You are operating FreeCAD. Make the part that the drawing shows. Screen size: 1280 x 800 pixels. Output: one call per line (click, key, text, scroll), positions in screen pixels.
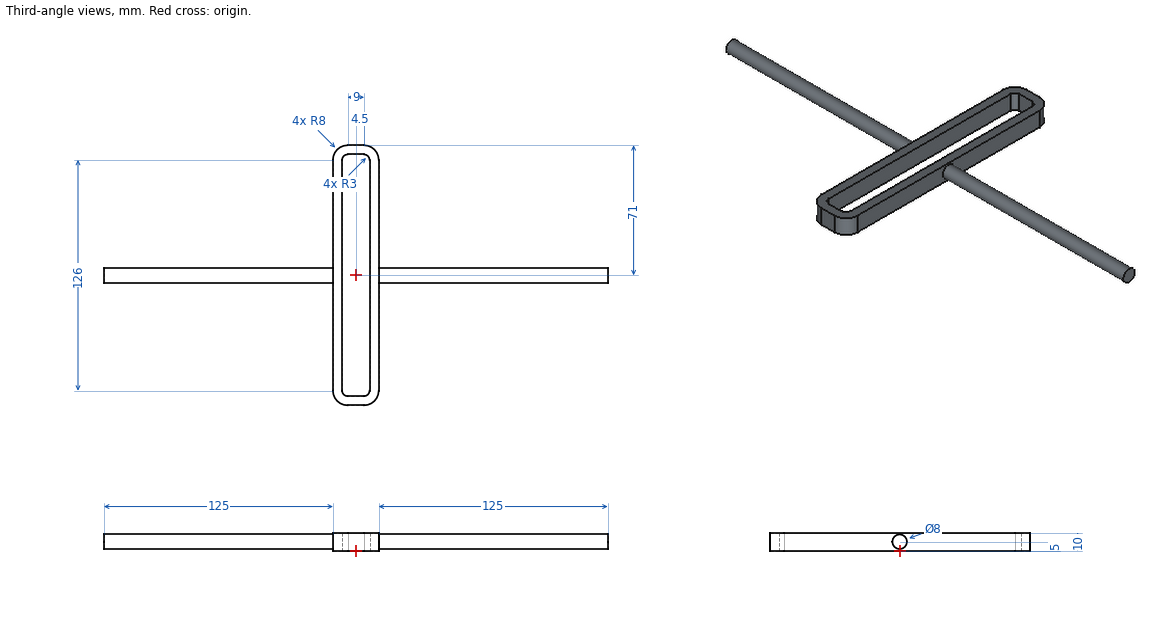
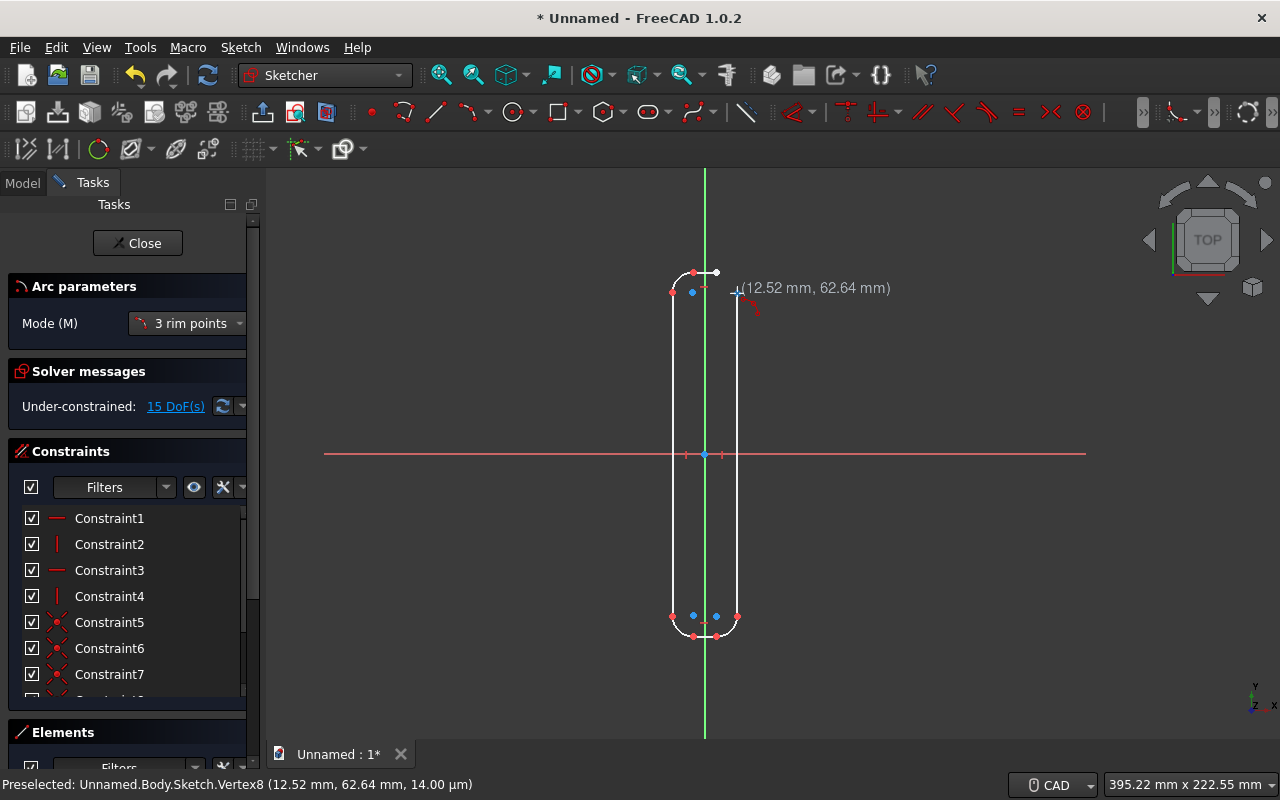
scroll(717, 272, up, 2)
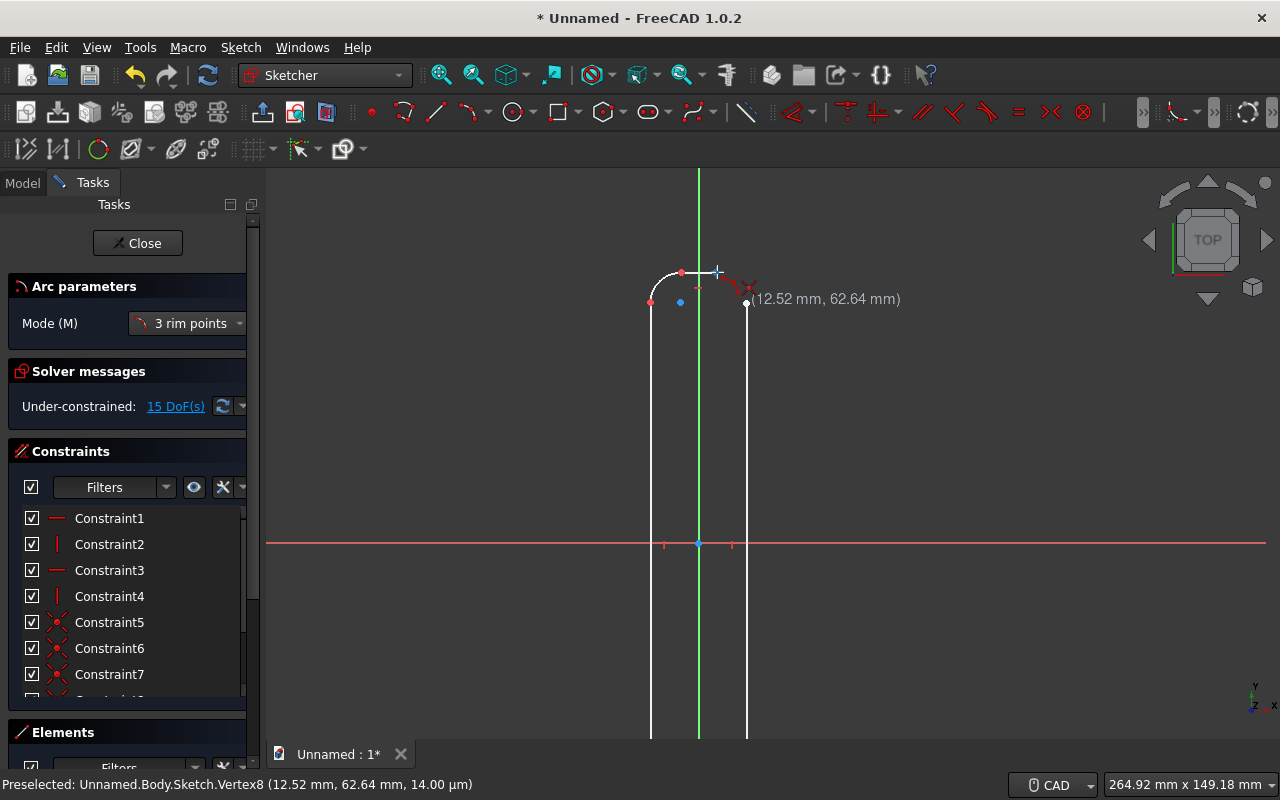
click(716, 273)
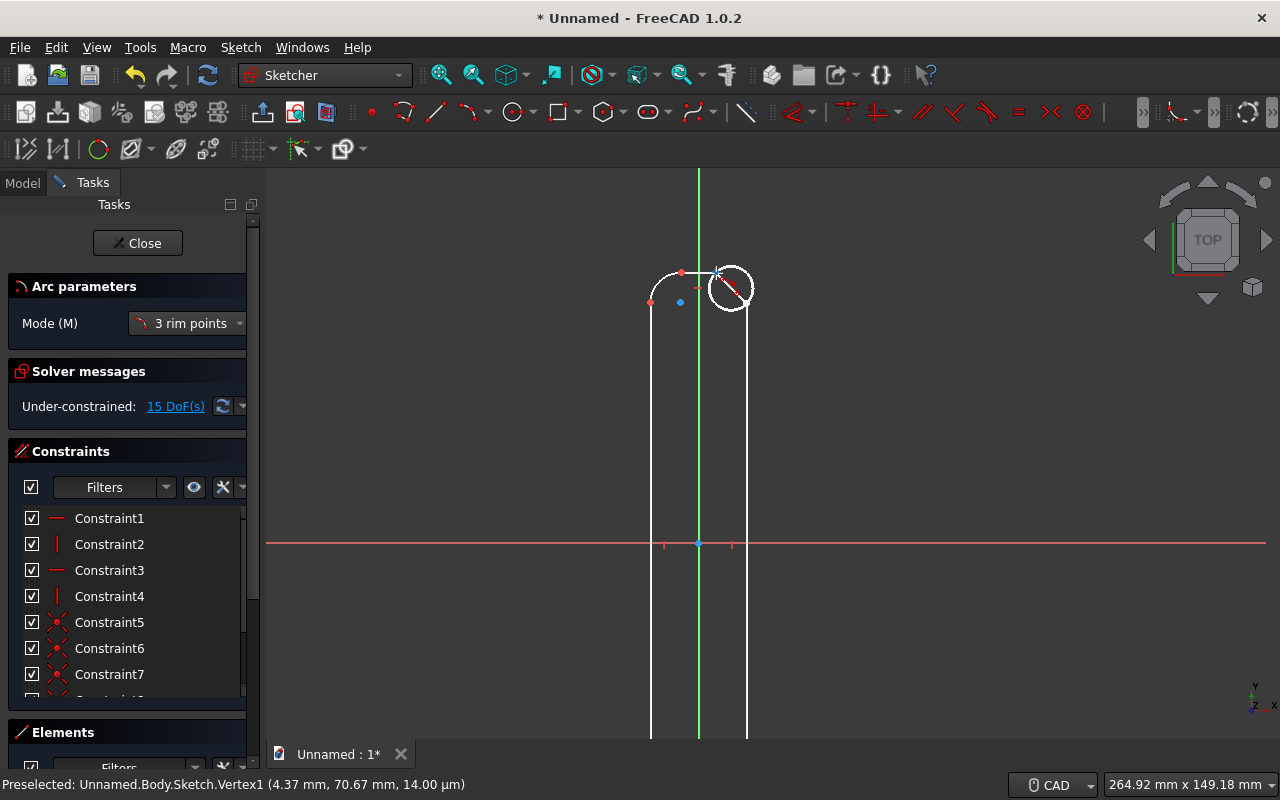
scroll(738, 281, up, 3)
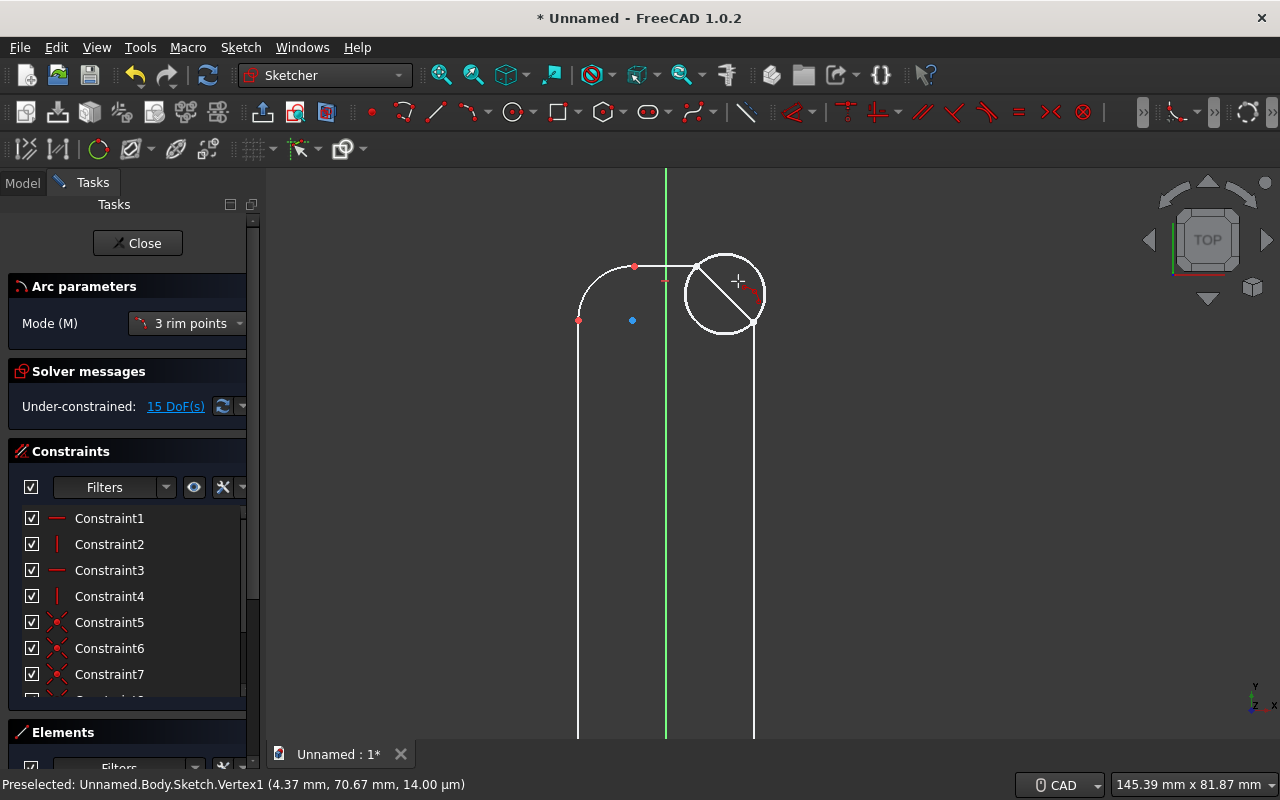
click(737, 280)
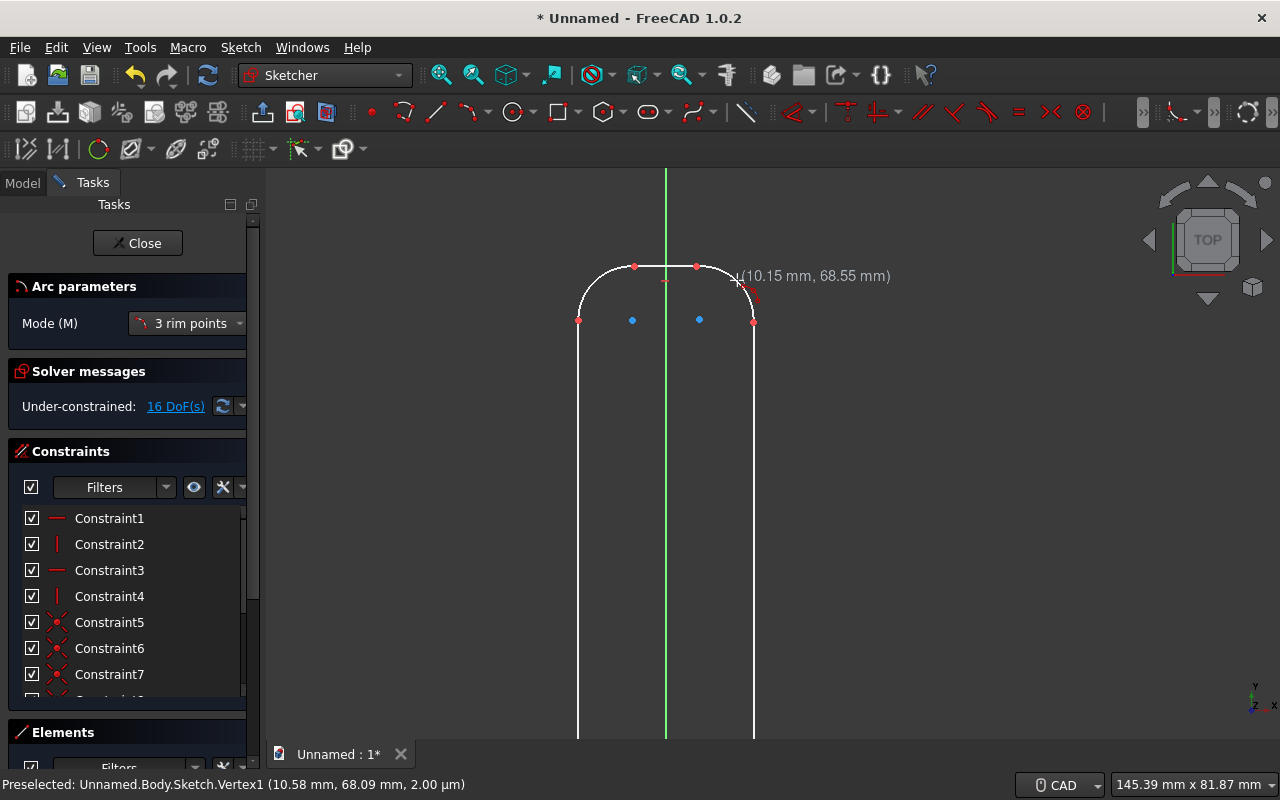
click(436, 112)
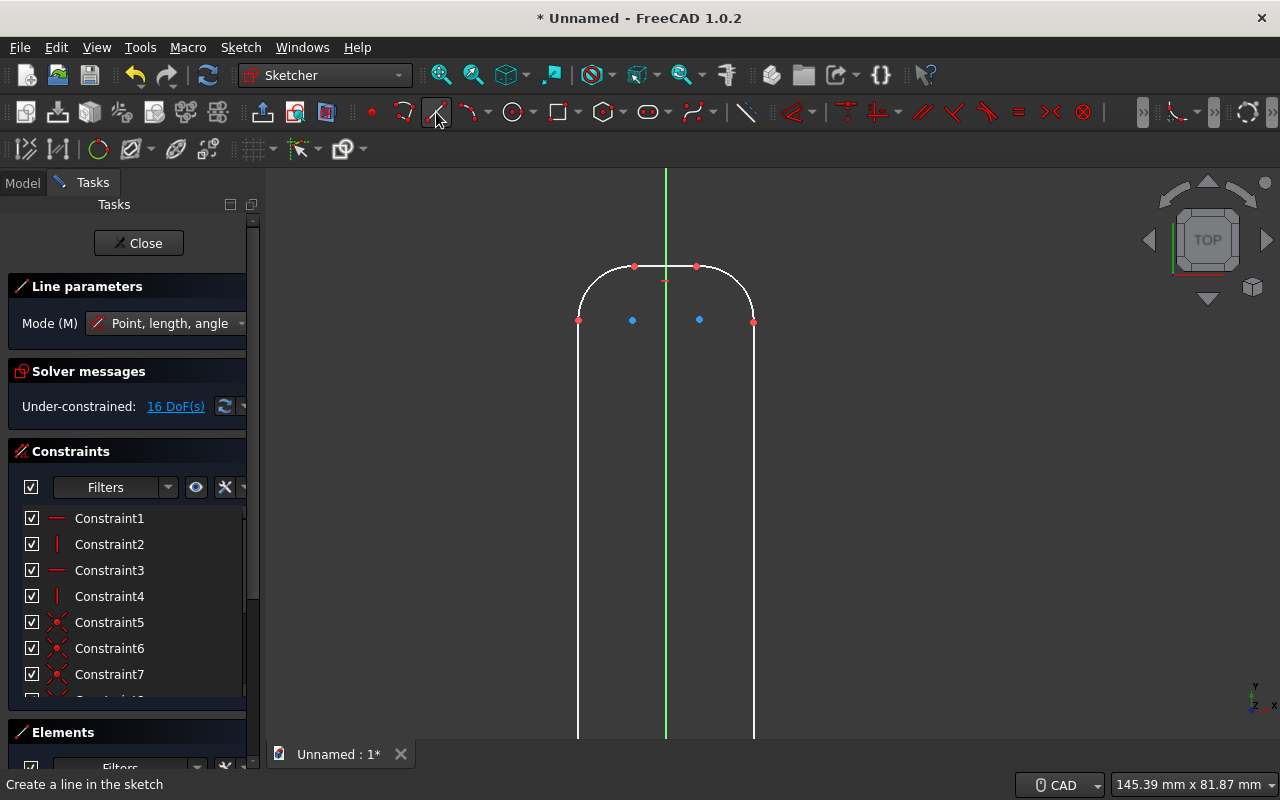
click(635, 299)
click(698, 299)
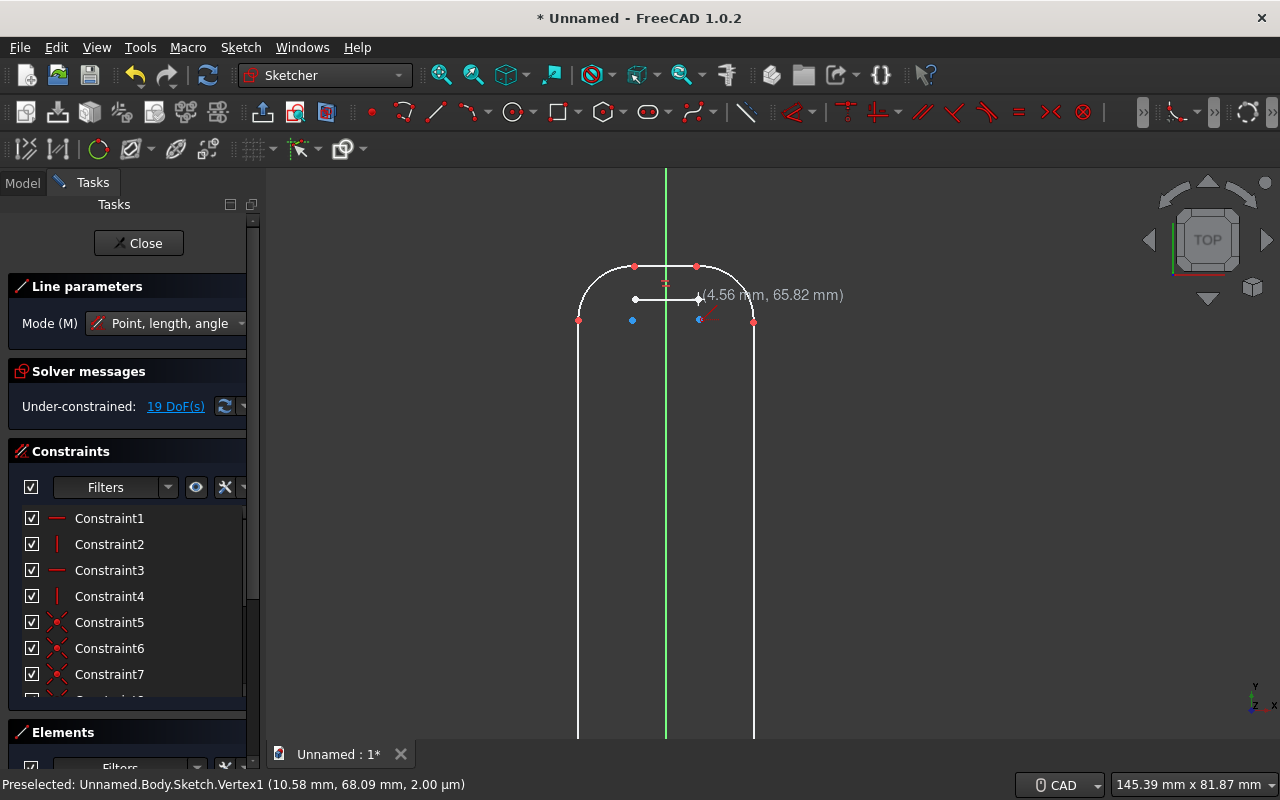
click(719, 320)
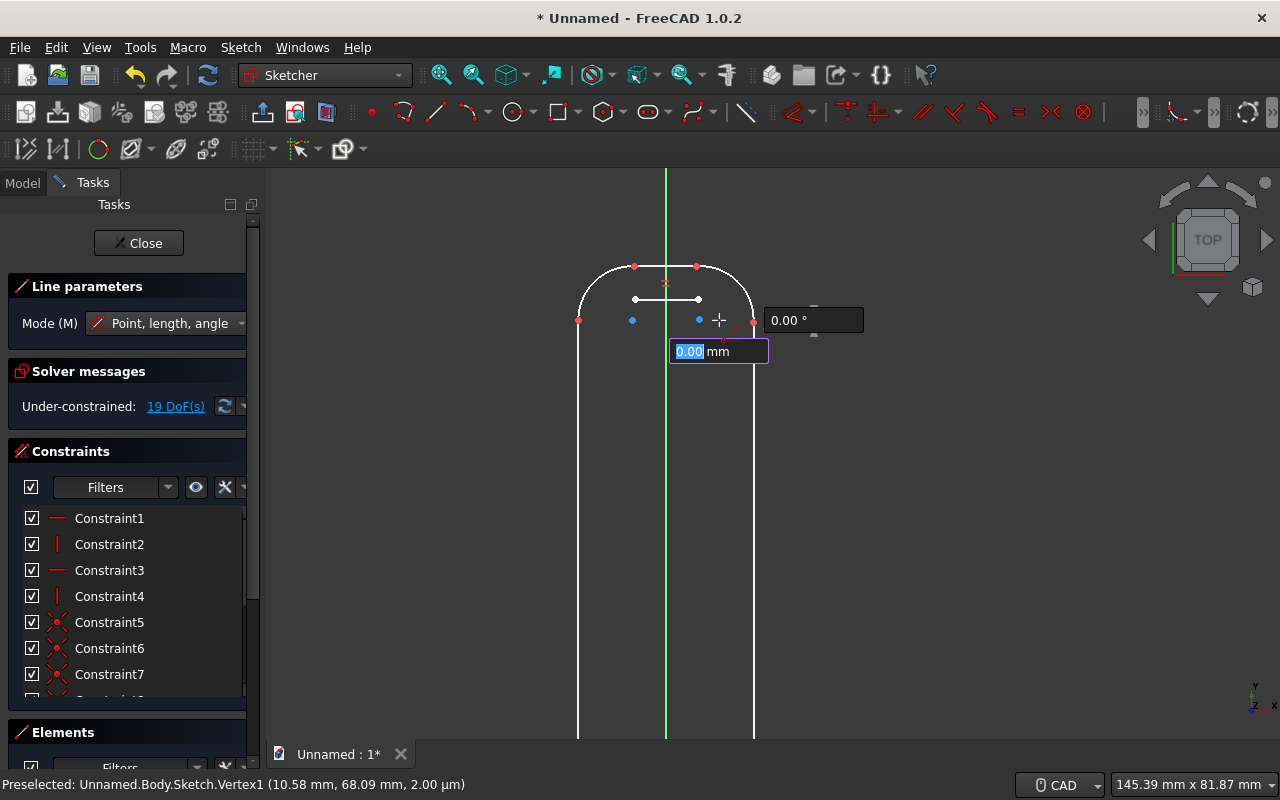
scroll(727, 276, down, 5)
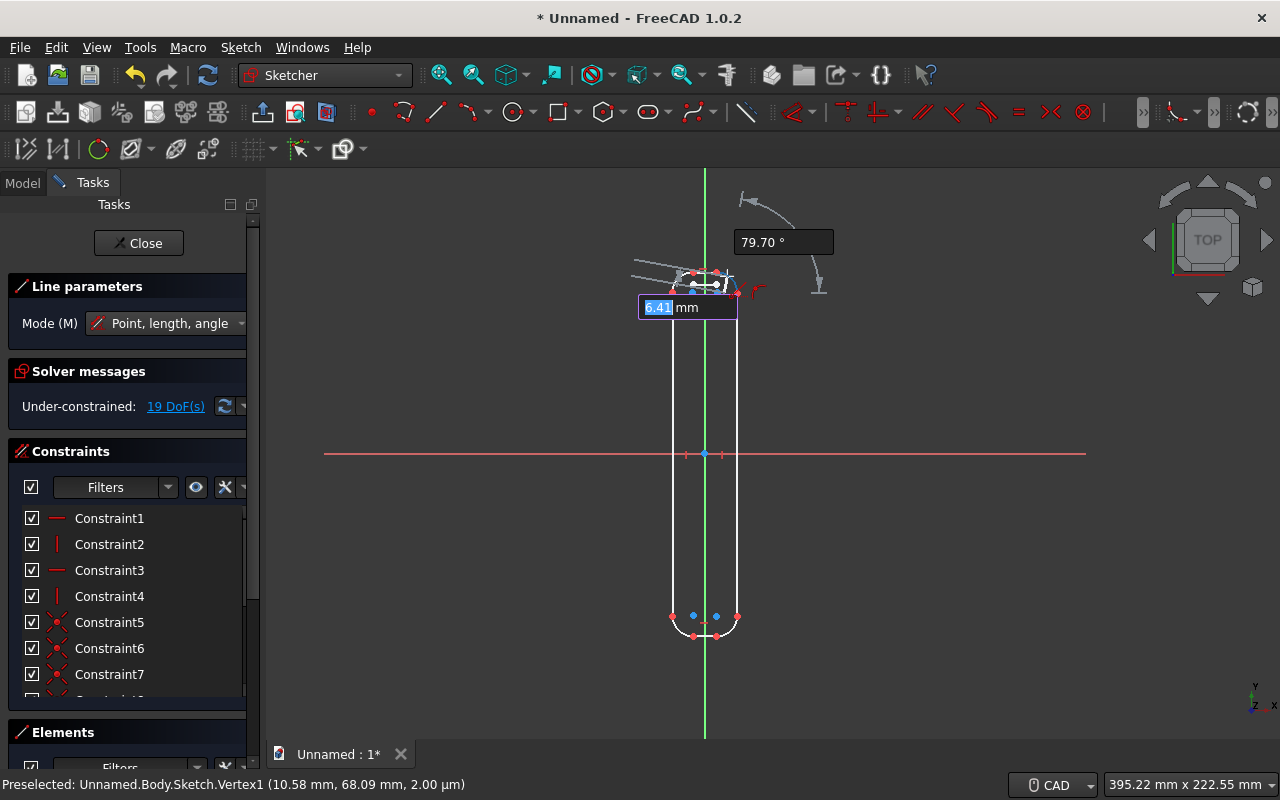
scroll(724, 615, up, 4)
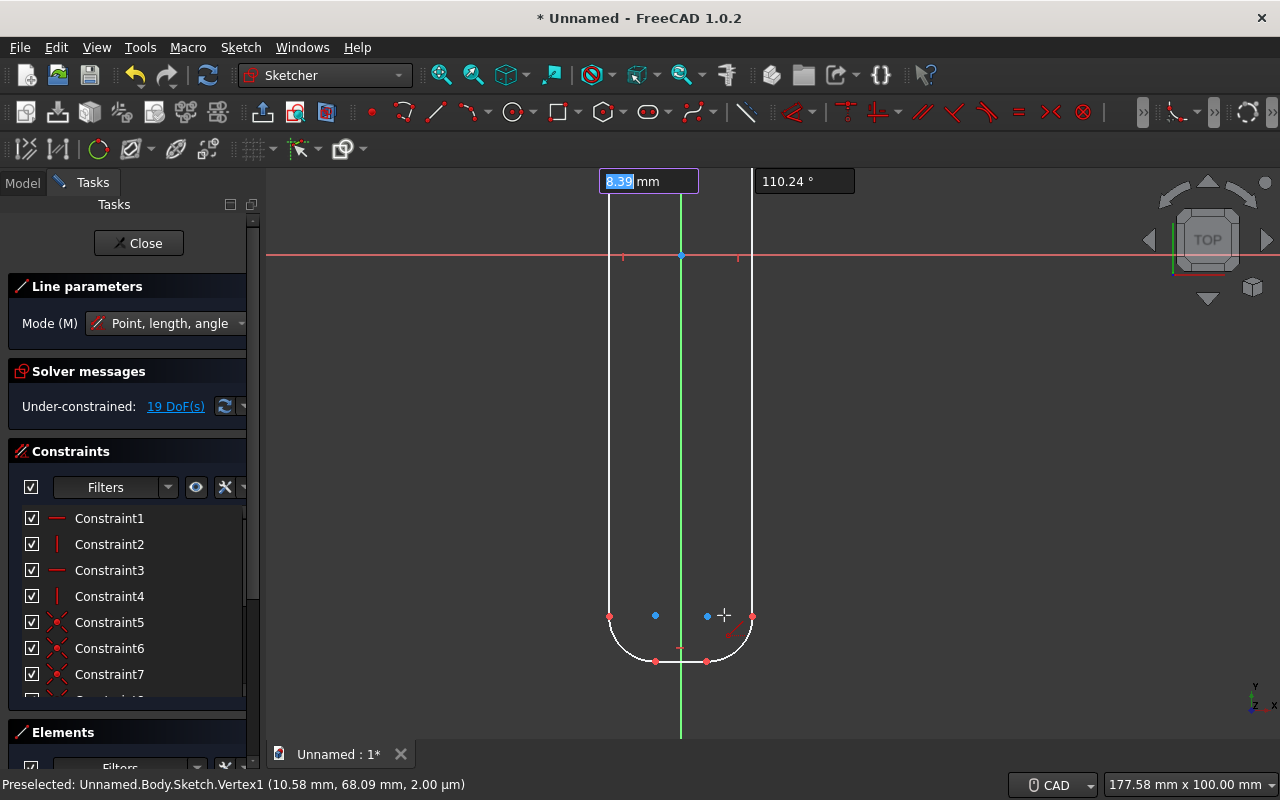
click(724, 615)